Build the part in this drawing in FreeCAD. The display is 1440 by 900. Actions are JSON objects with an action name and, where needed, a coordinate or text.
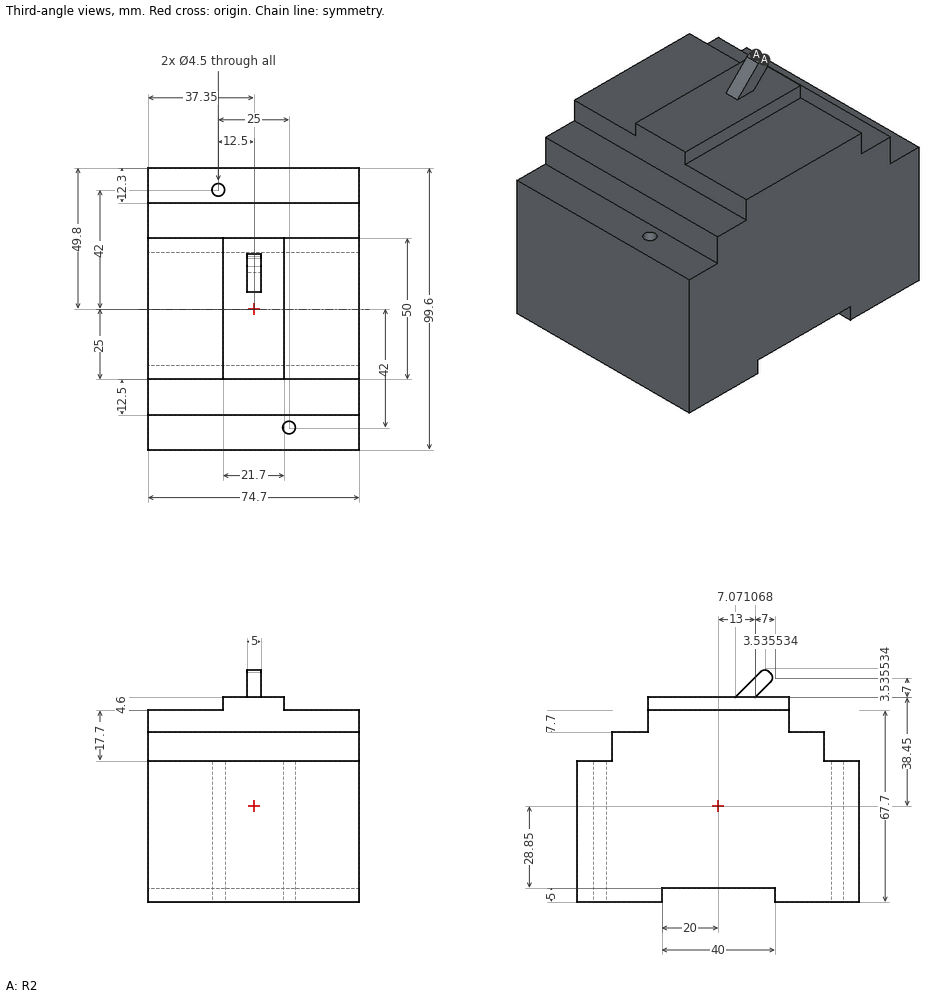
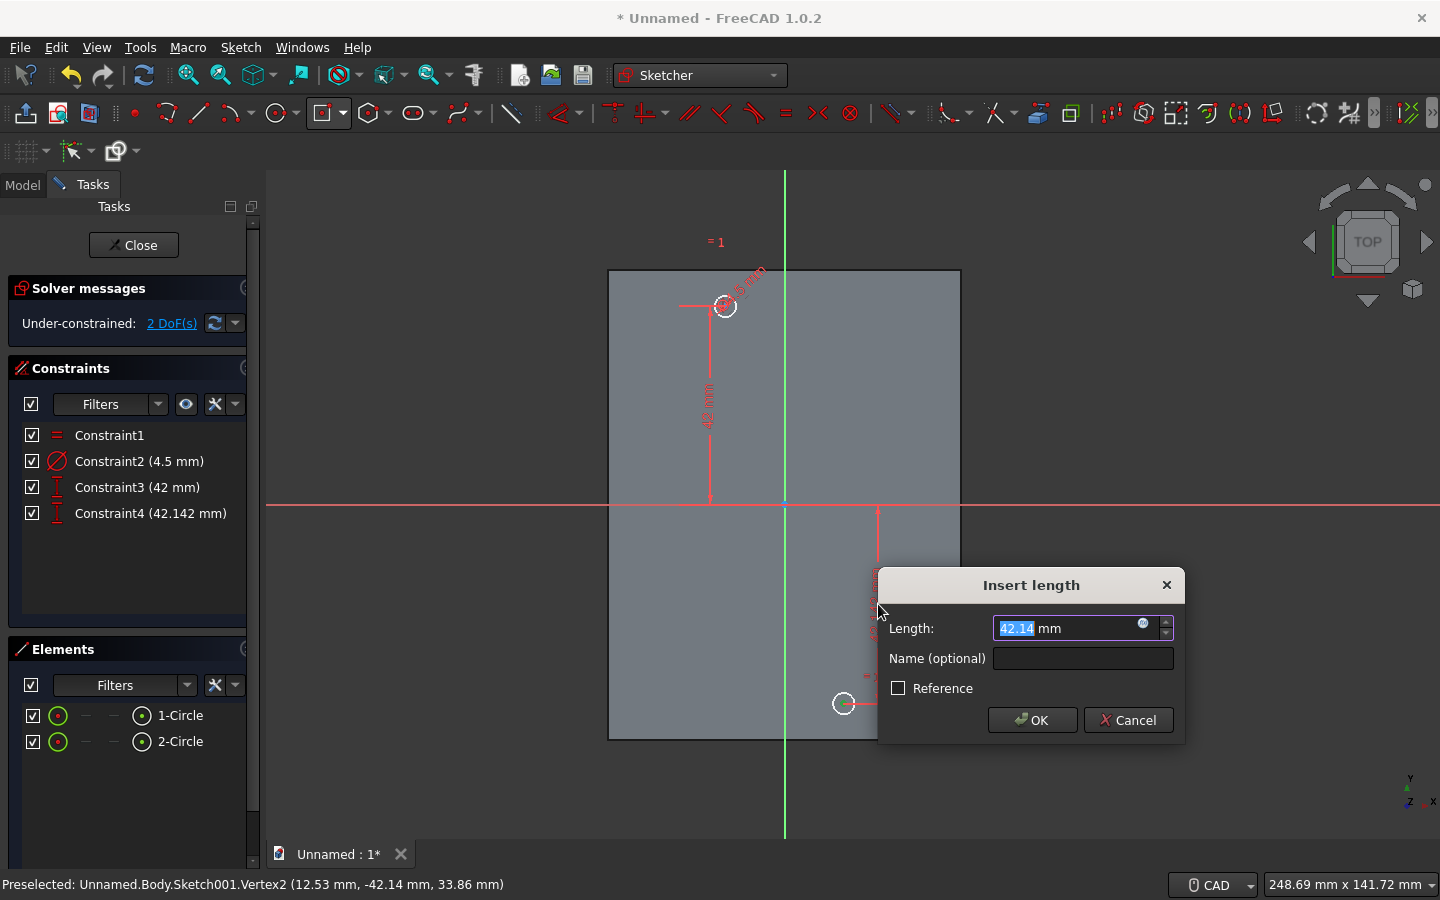
{"action": "type", "text": "42"}
{"action": "key", "text": "Return"}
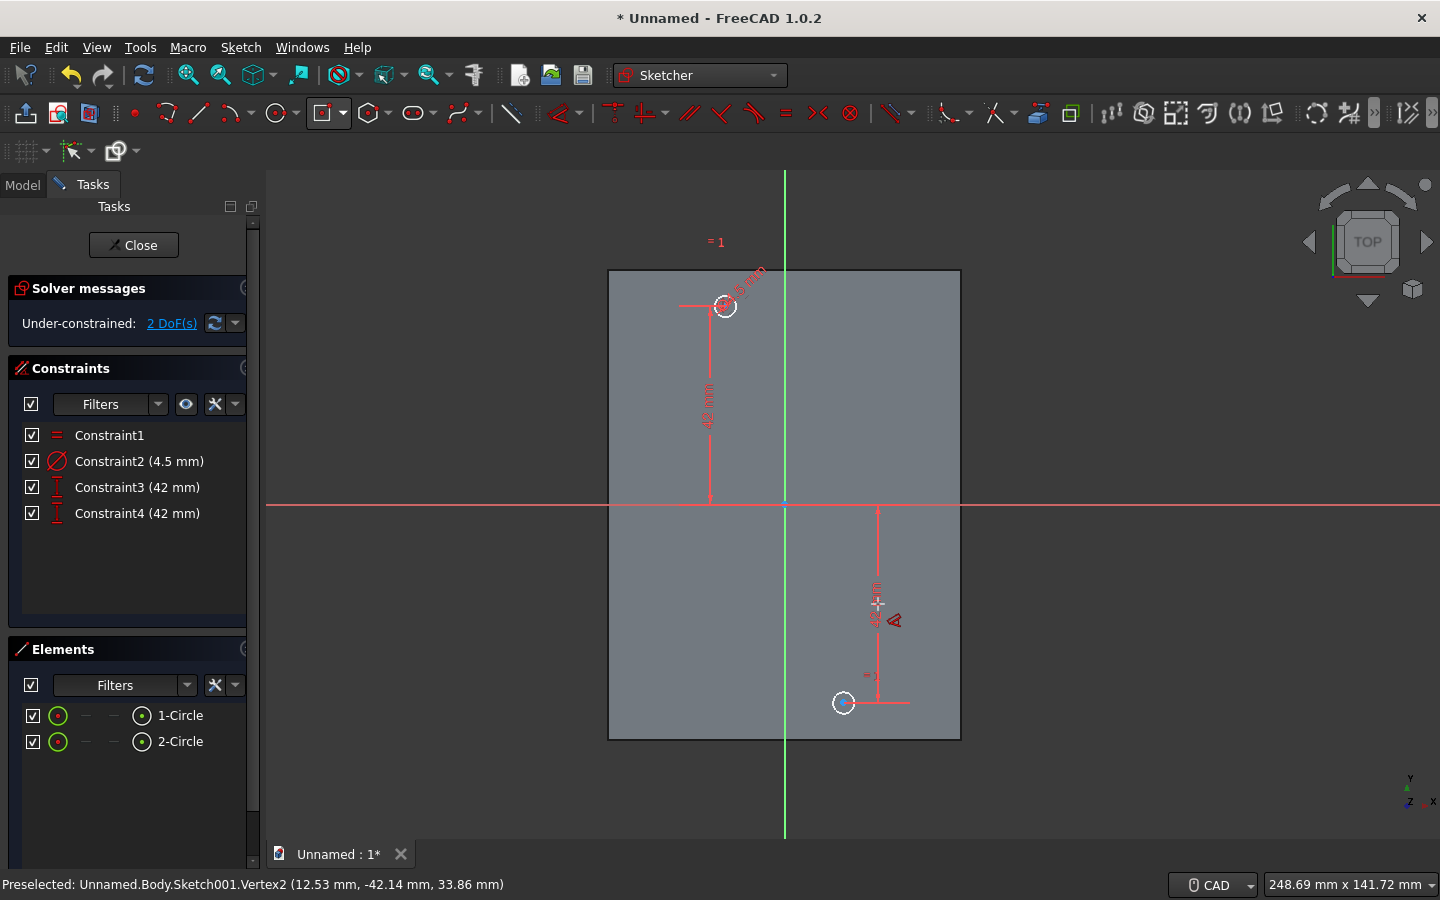
{"action": "left_click", "coordinate": [725, 306]}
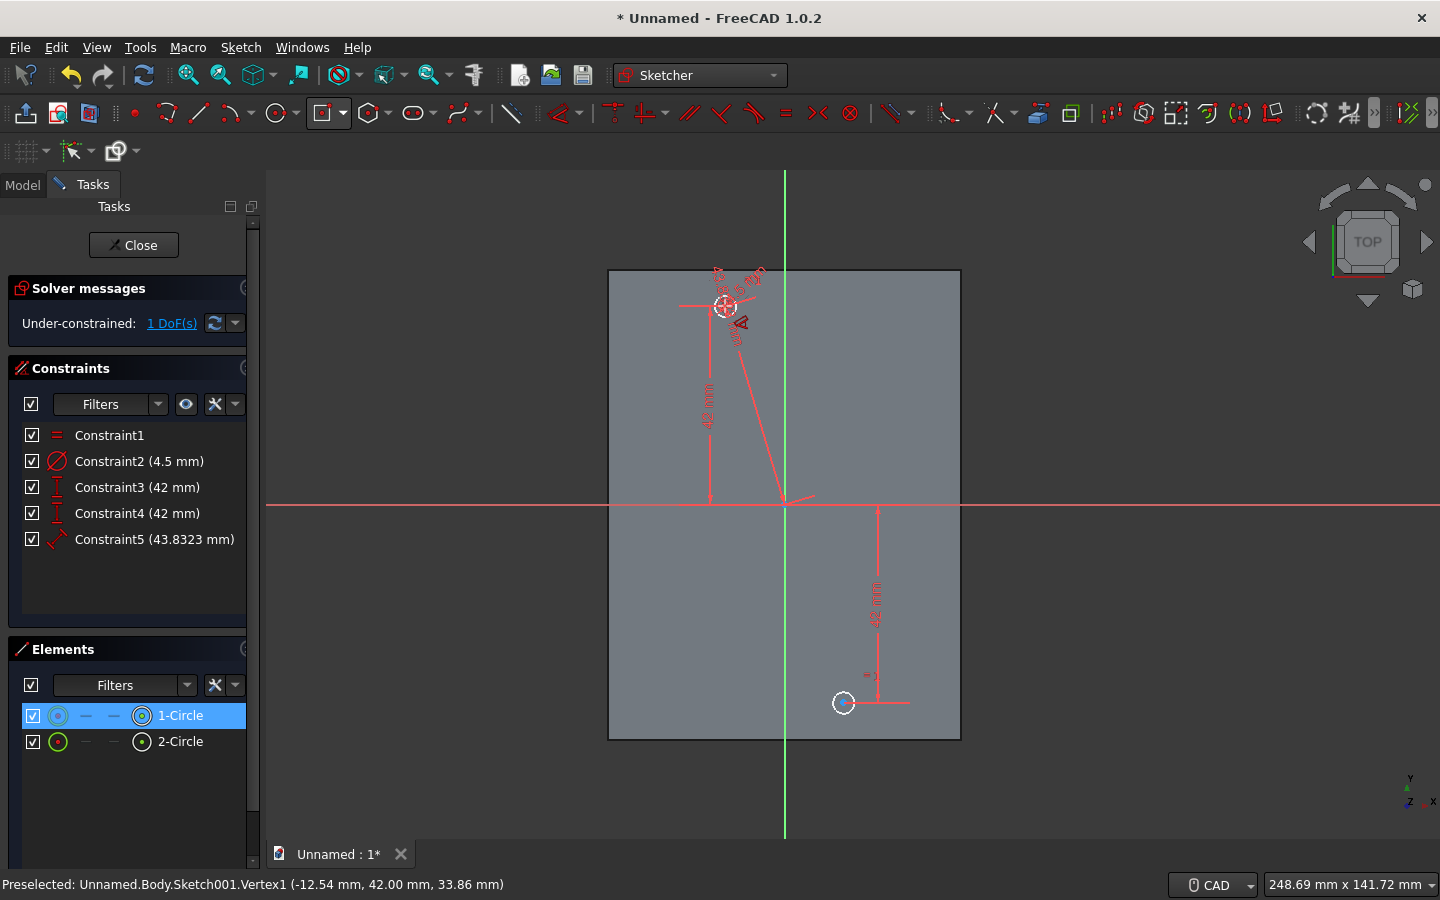
{"action": "left_click", "coordinate": [844, 703]}
{"action": "left_click", "coordinate": [757, 737]}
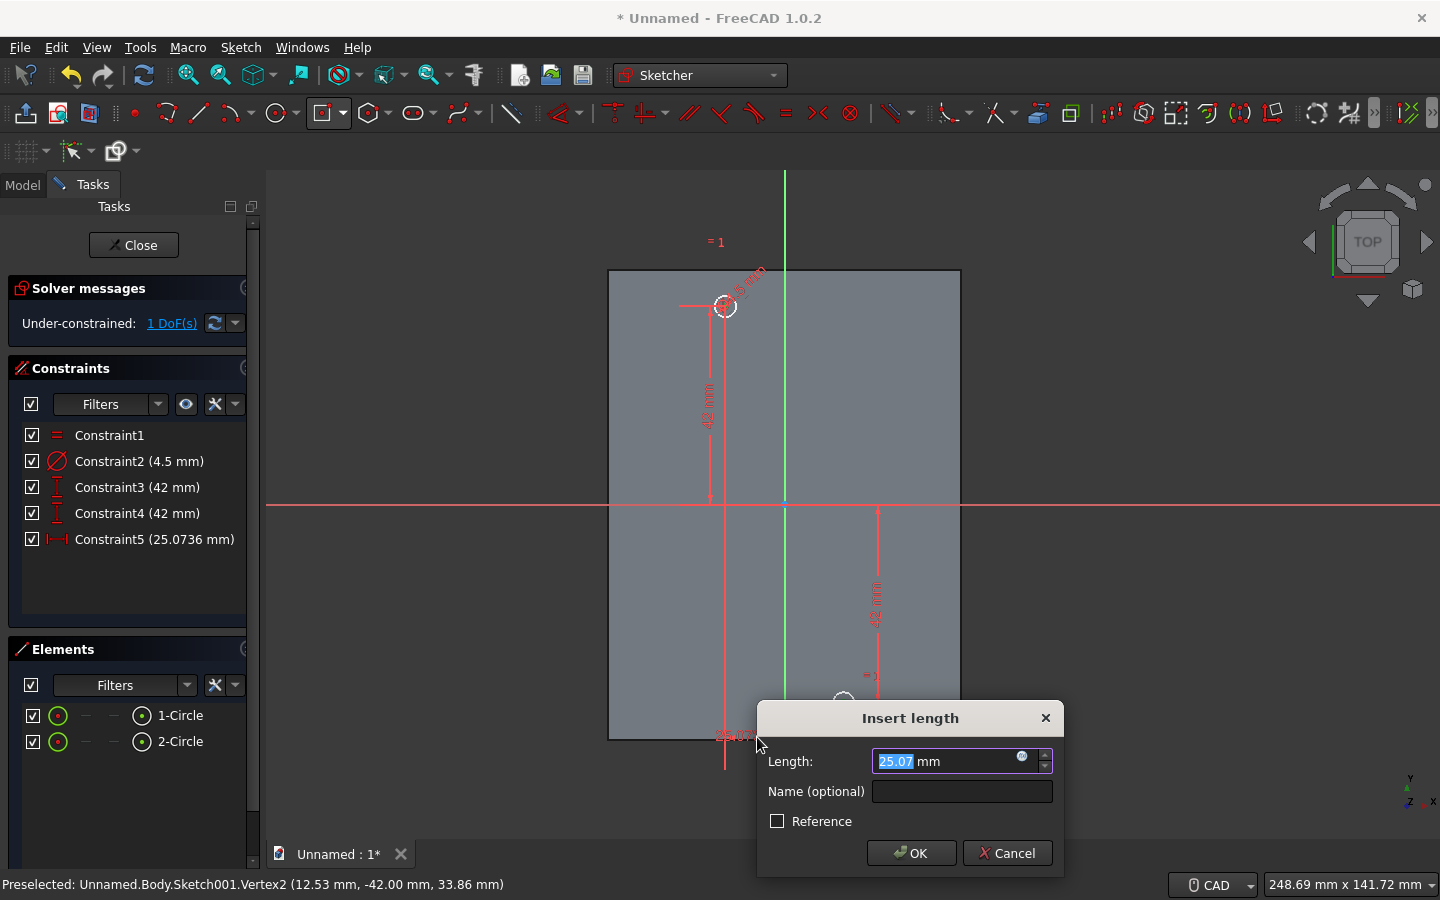
{"action": "type", "text": "25"}
{"action": "key", "text": "Return"}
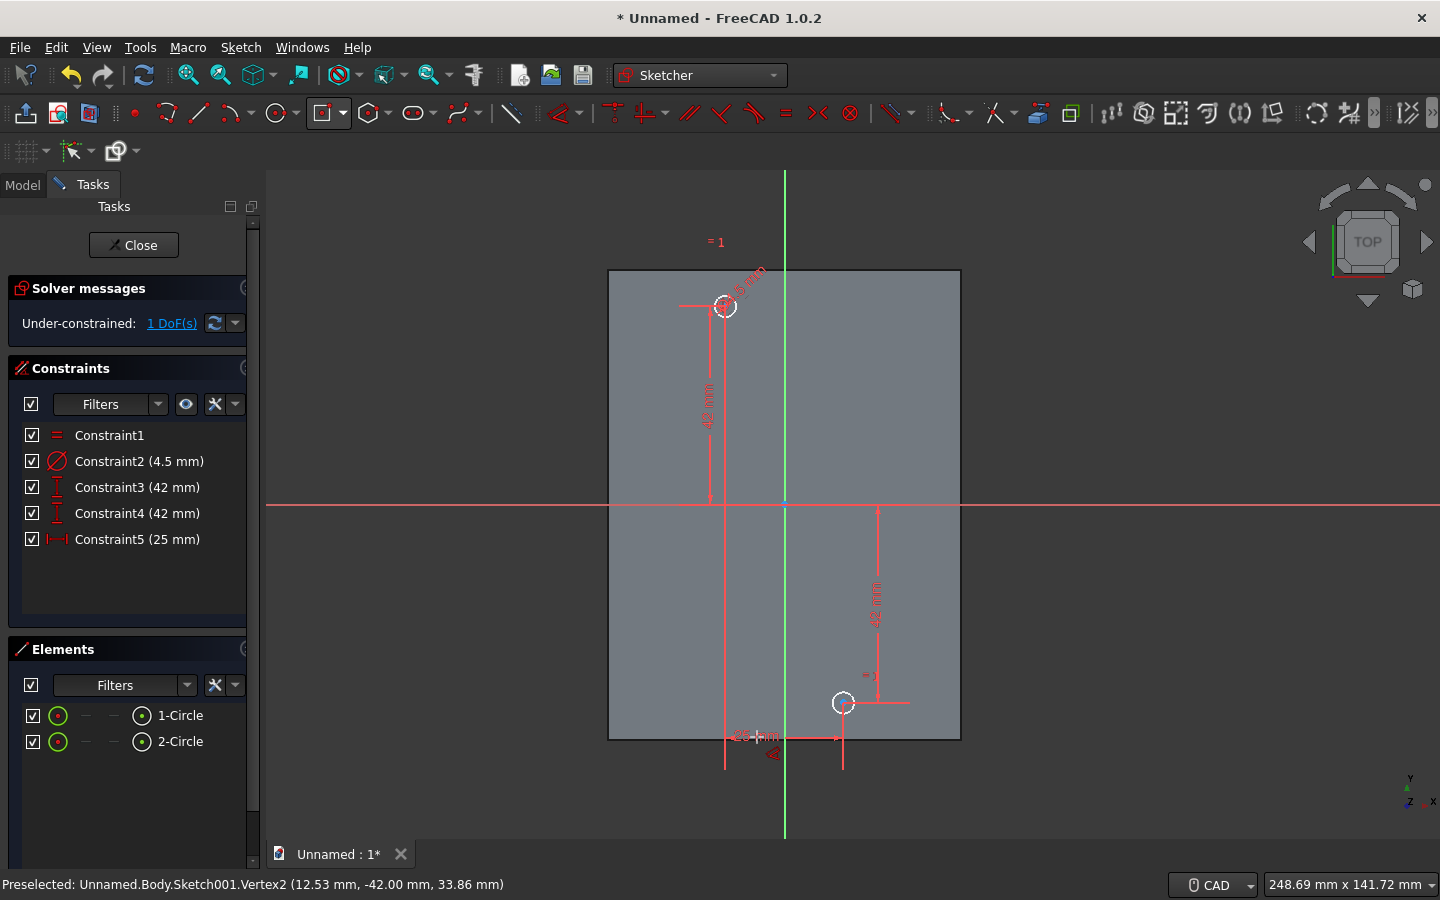
{"action": "left_click", "coordinate": [725, 306]}
{"action": "left_click", "coordinate": [755, 539]}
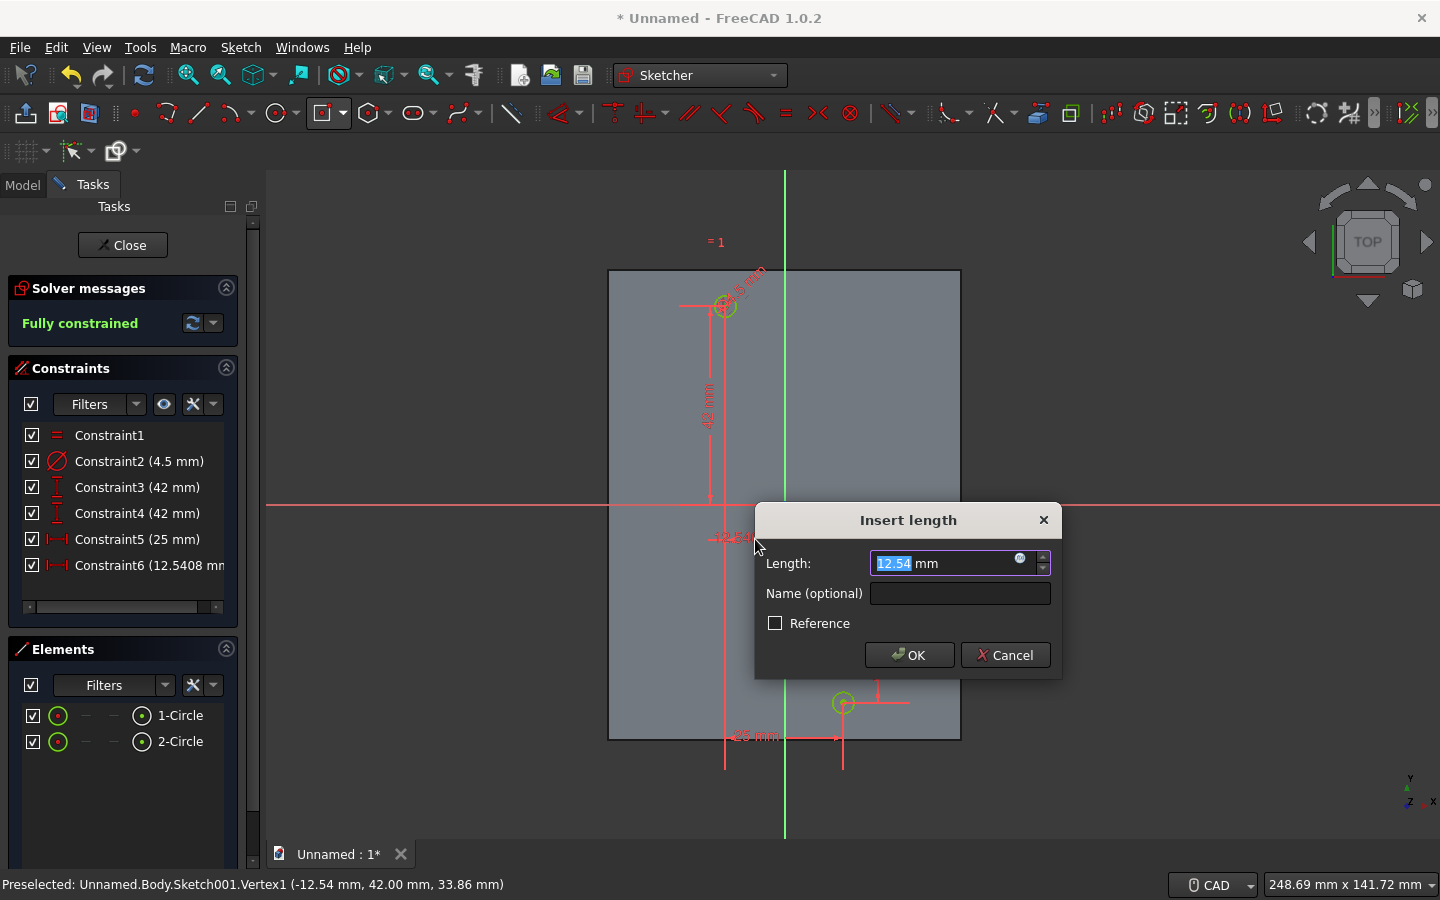
{"action": "type", "text": "12.5"}
{"action": "key", "text": "Return"}
{"action": "key", "text": "Escape"}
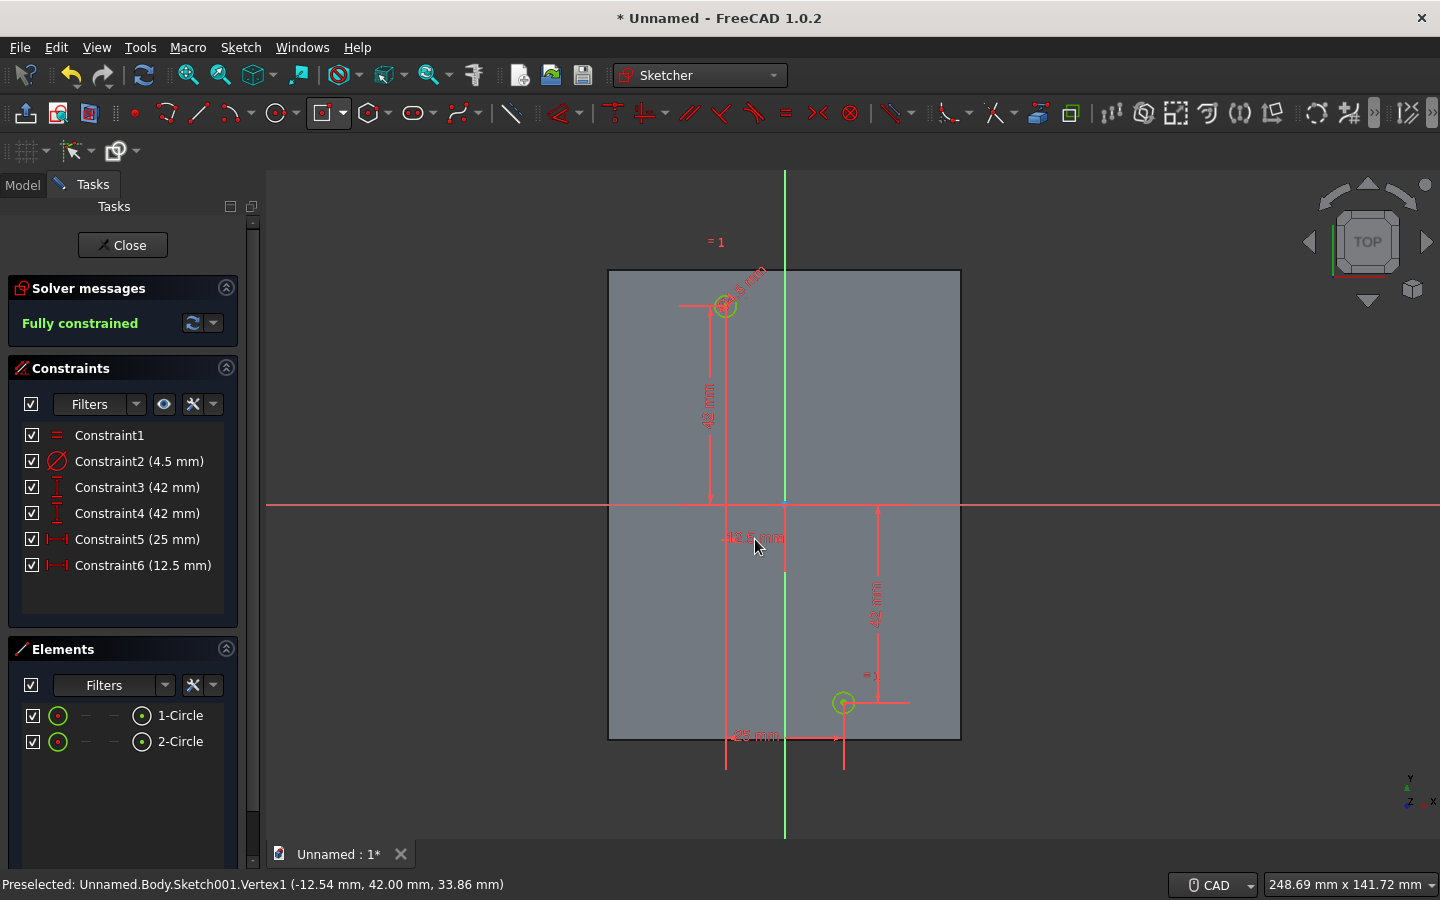
{"action": "left_click", "coordinate": [123, 245]}